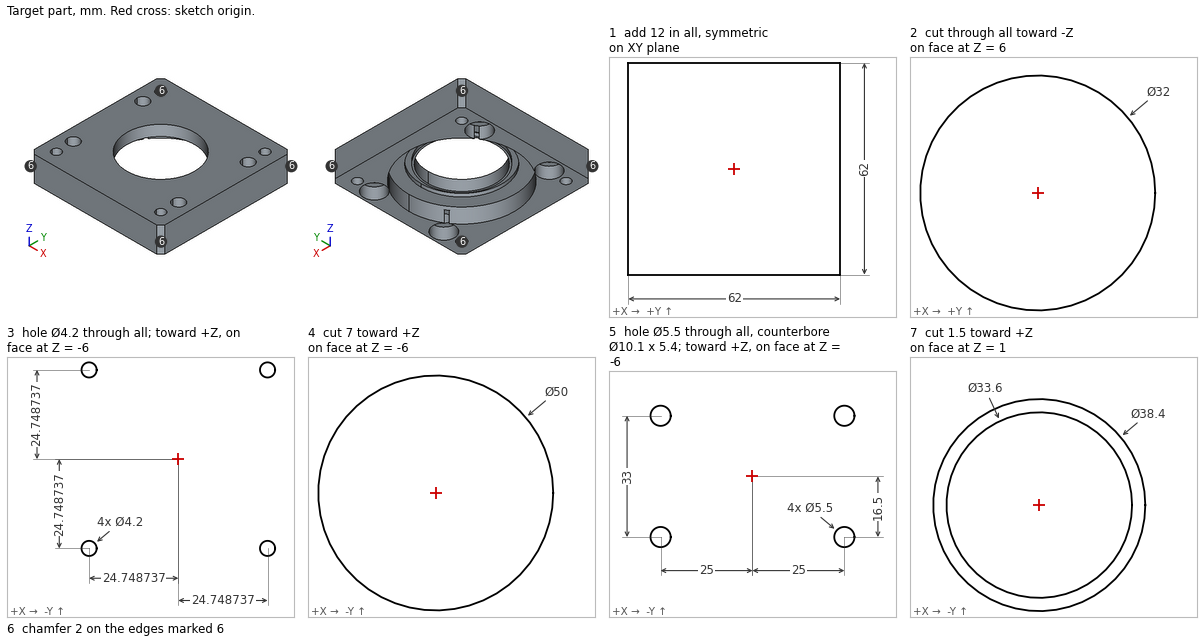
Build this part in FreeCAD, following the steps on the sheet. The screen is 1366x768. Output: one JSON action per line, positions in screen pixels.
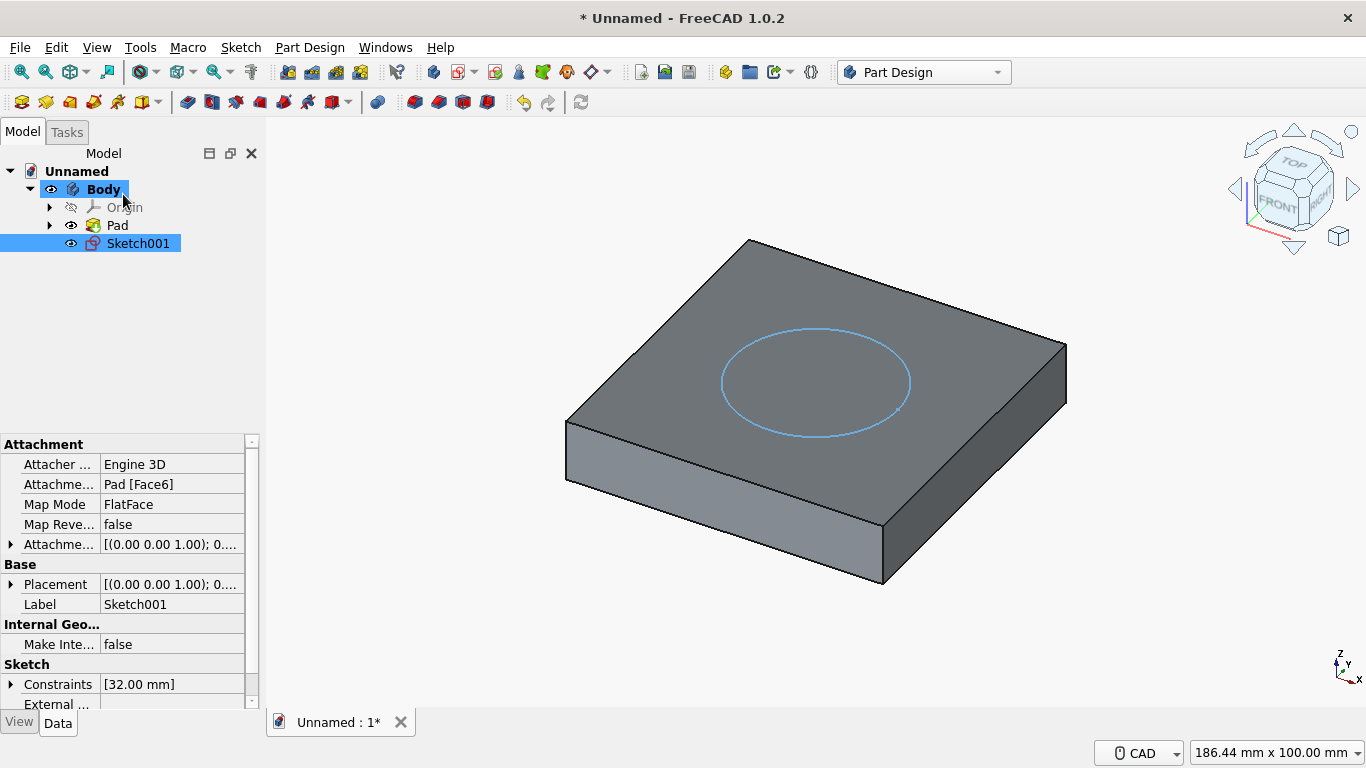
{"action": "left_click", "coordinate": [188, 102]}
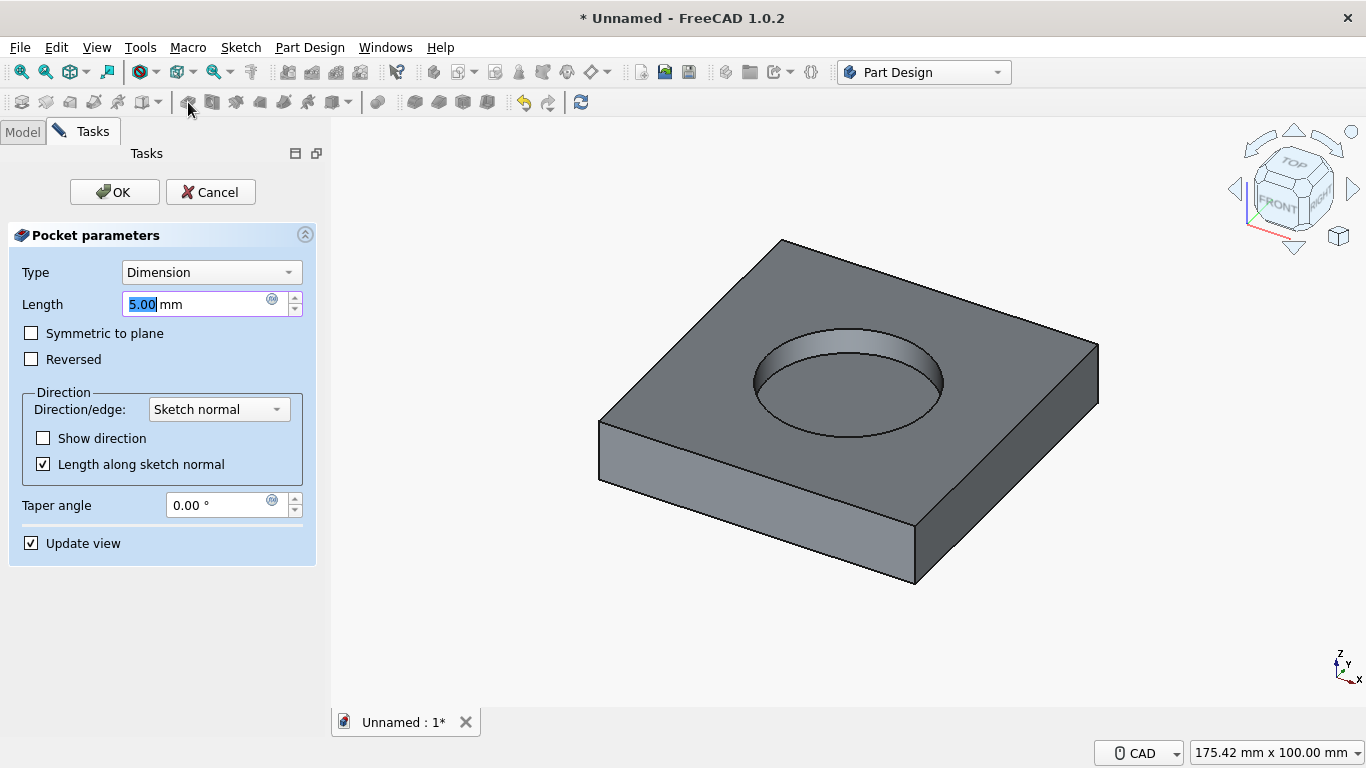
{"action": "left_click", "coordinate": [212, 272]}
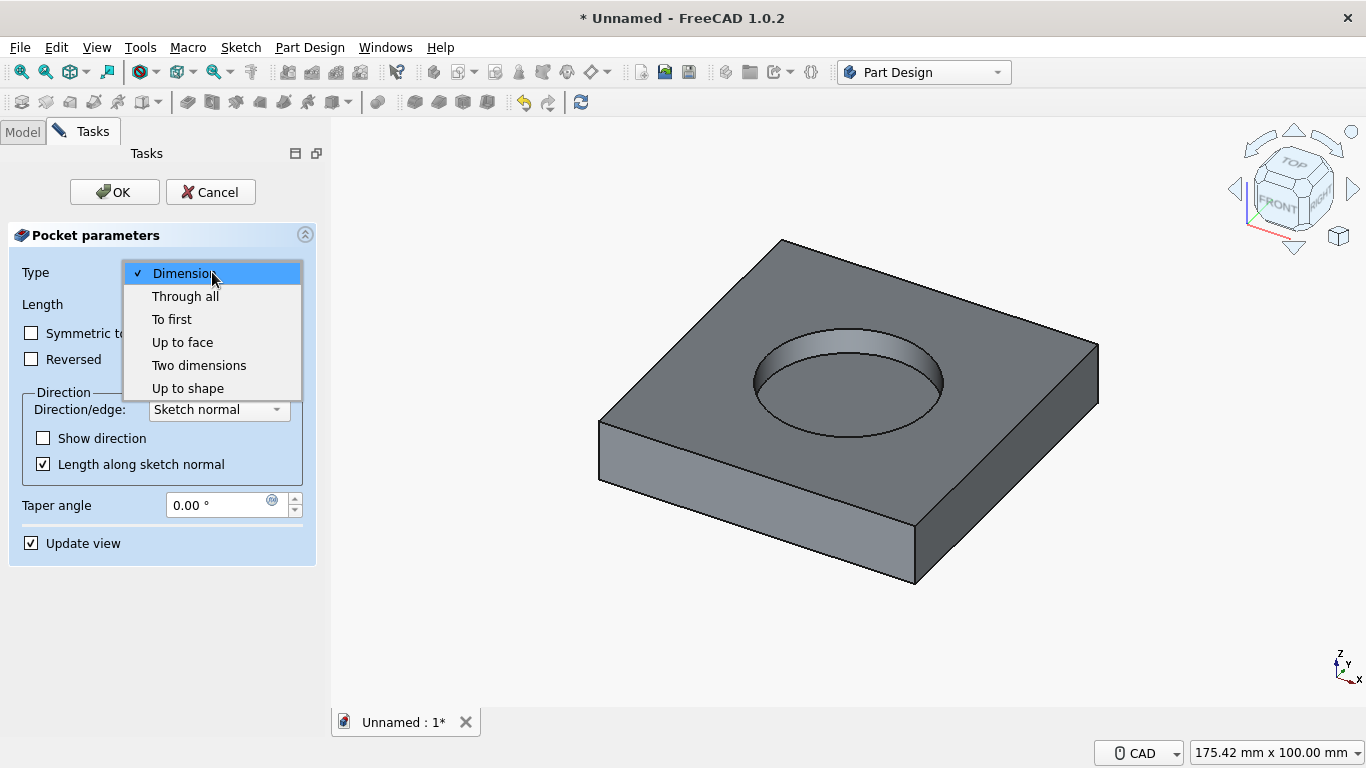
{"action": "left_click", "coordinate": [212, 296]}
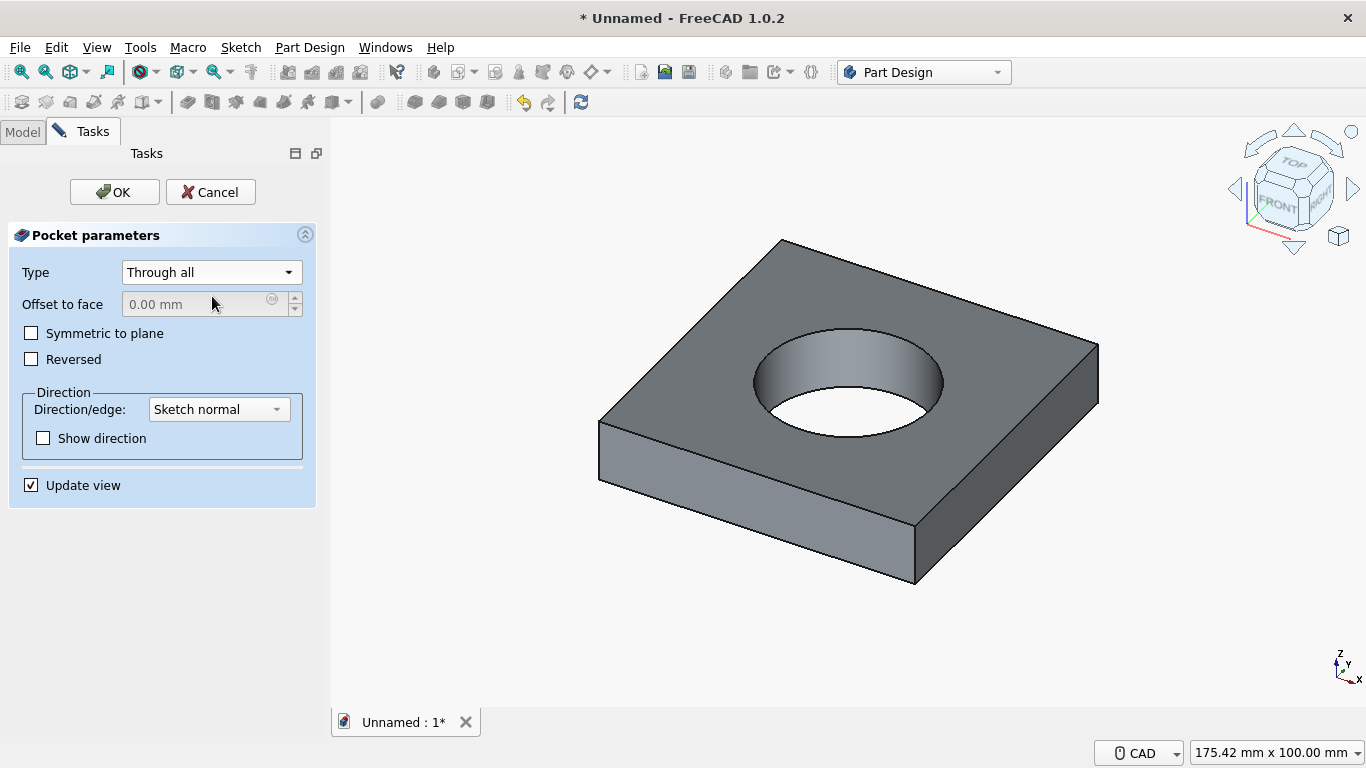
{"action": "left_click", "coordinate": [115, 192]}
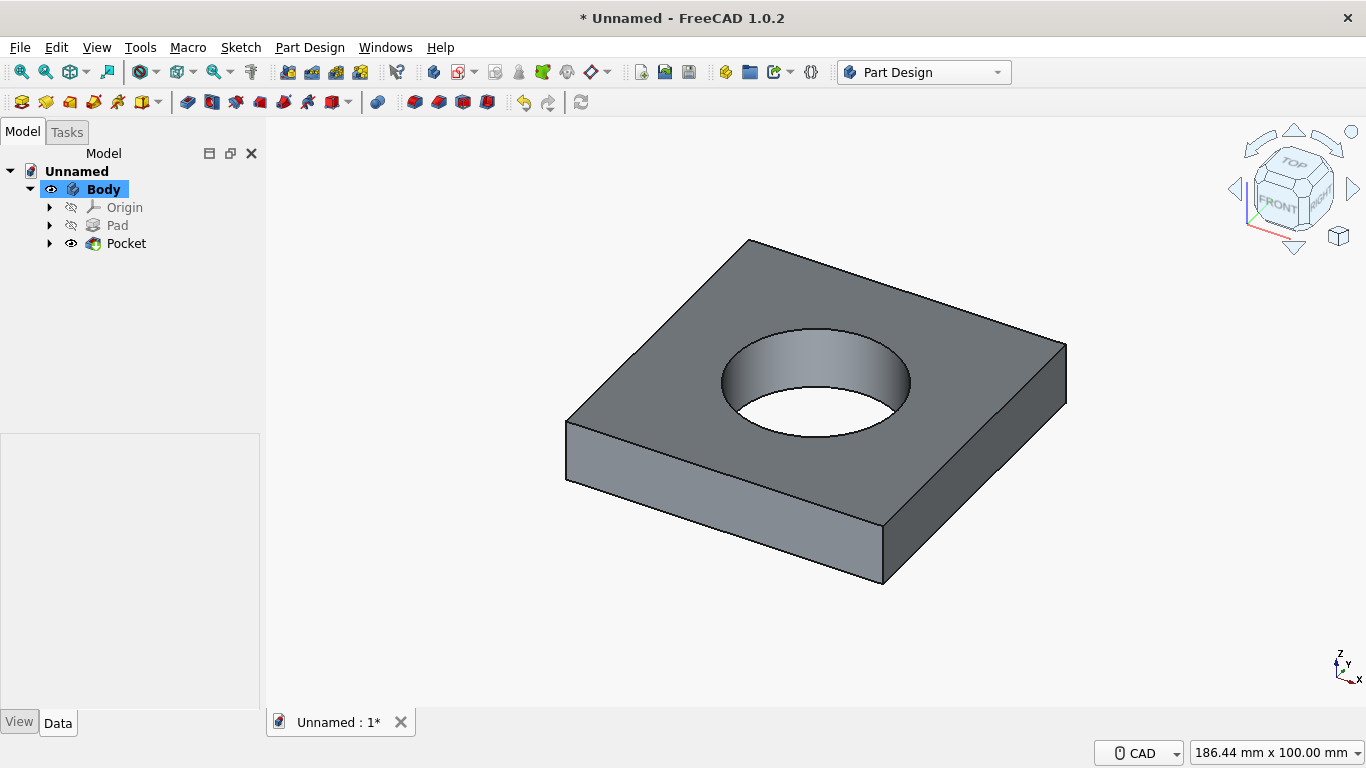
{"action": "key", "text": "5"}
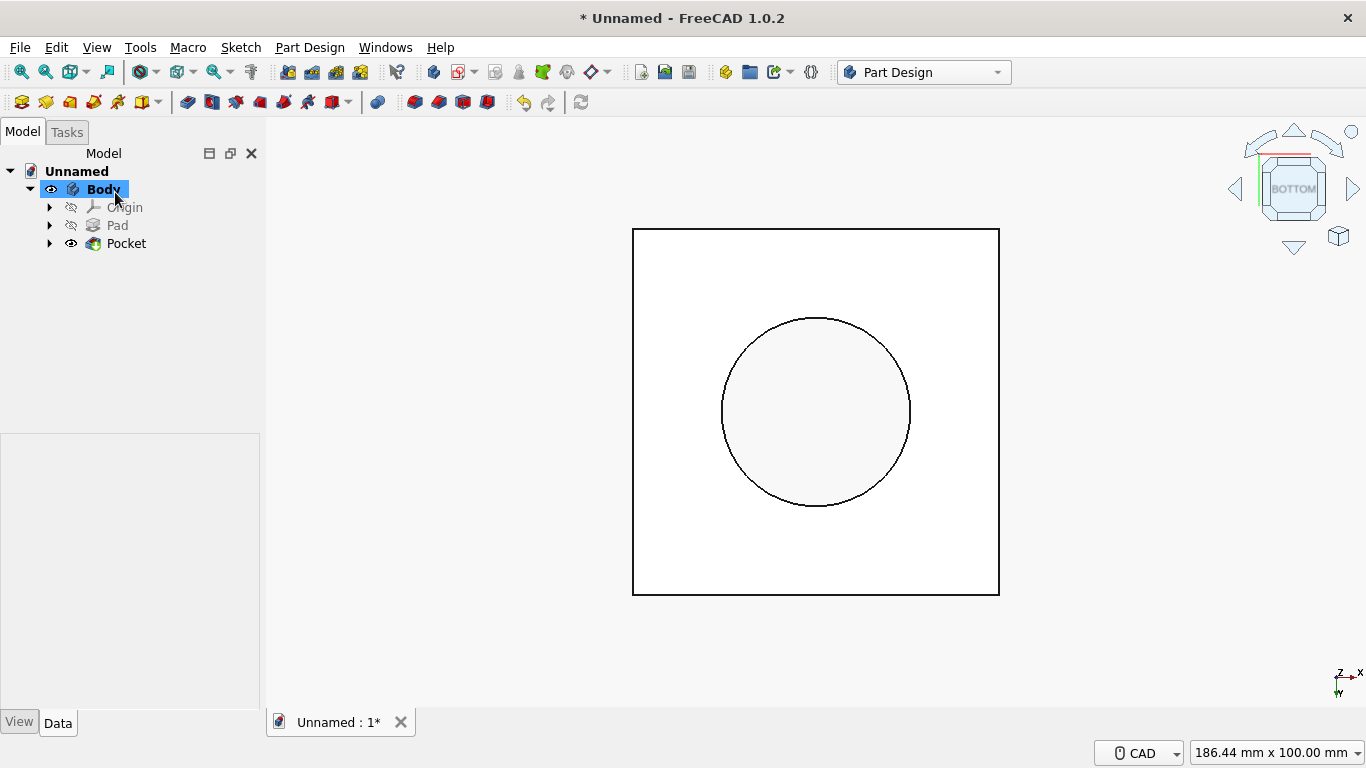
{"action": "left_click", "coordinate": [921, 516]}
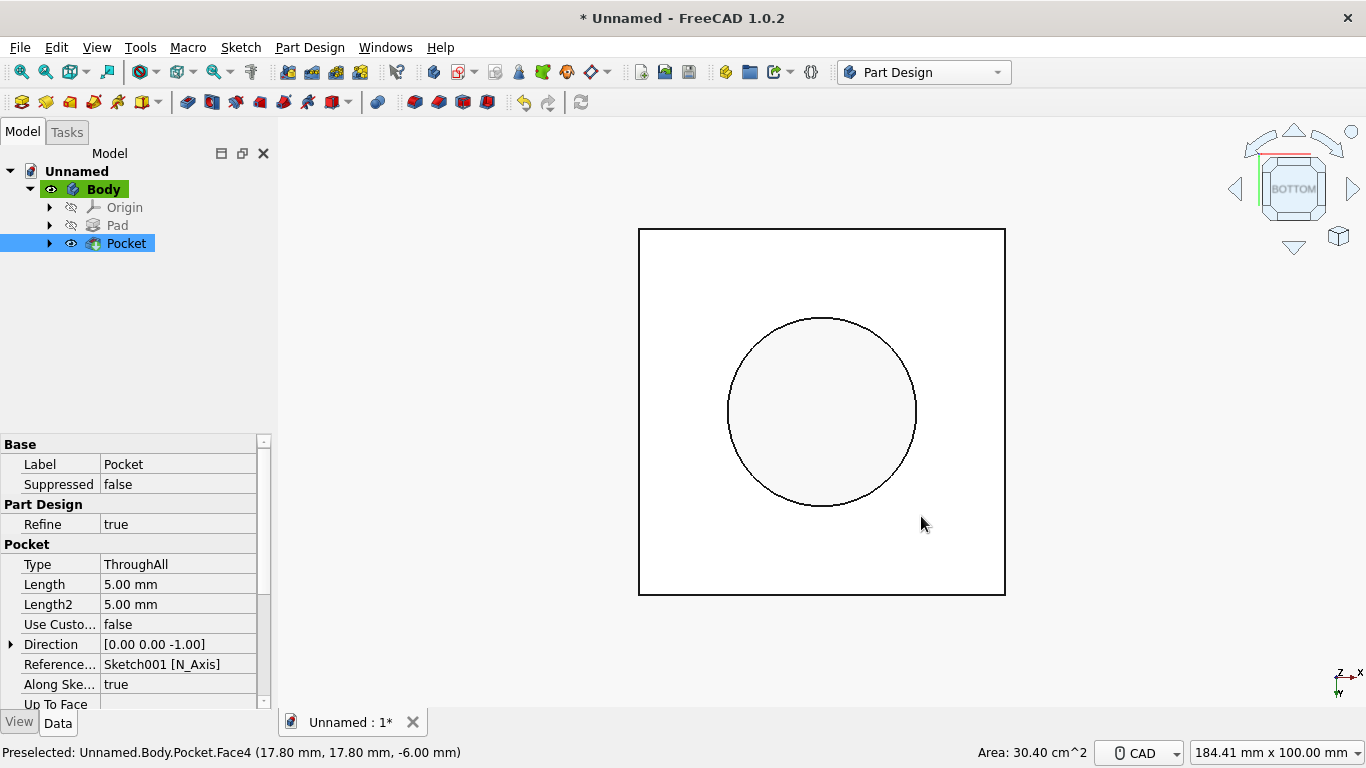
{"action": "left_click", "coordinate": [458, 72]}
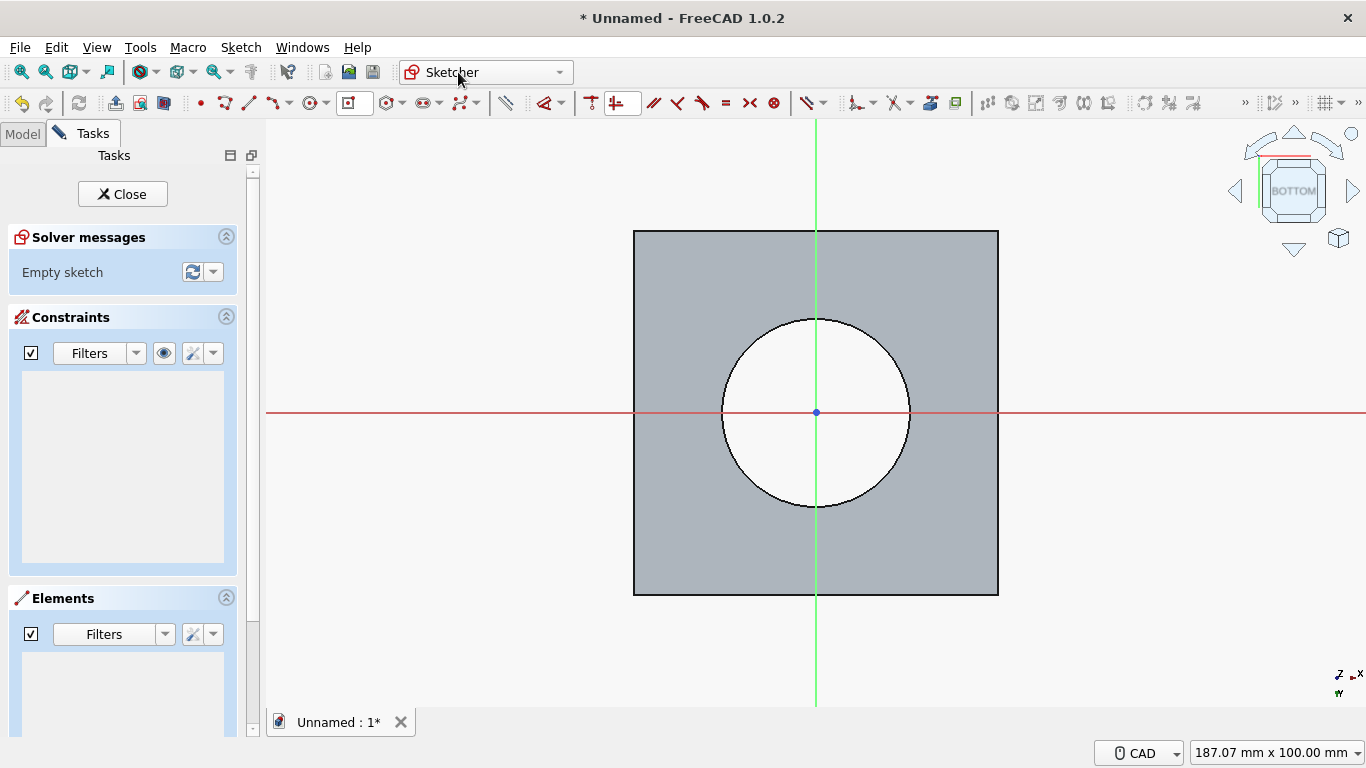
{"action": "left_click", "coordinate": [310, 104]}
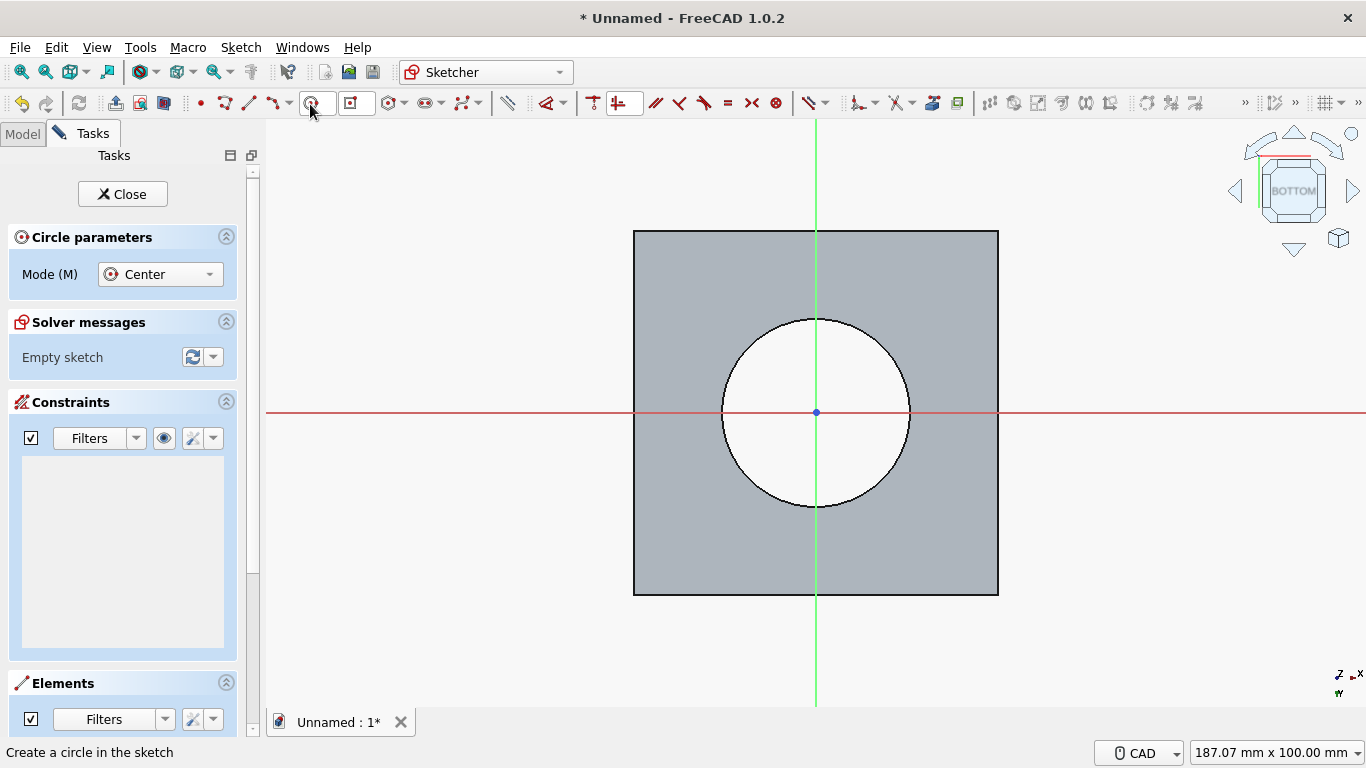
{"action": "scroll", "coordinate": [670, 559], "scroll_direction": "up", "scroll_amount": 4}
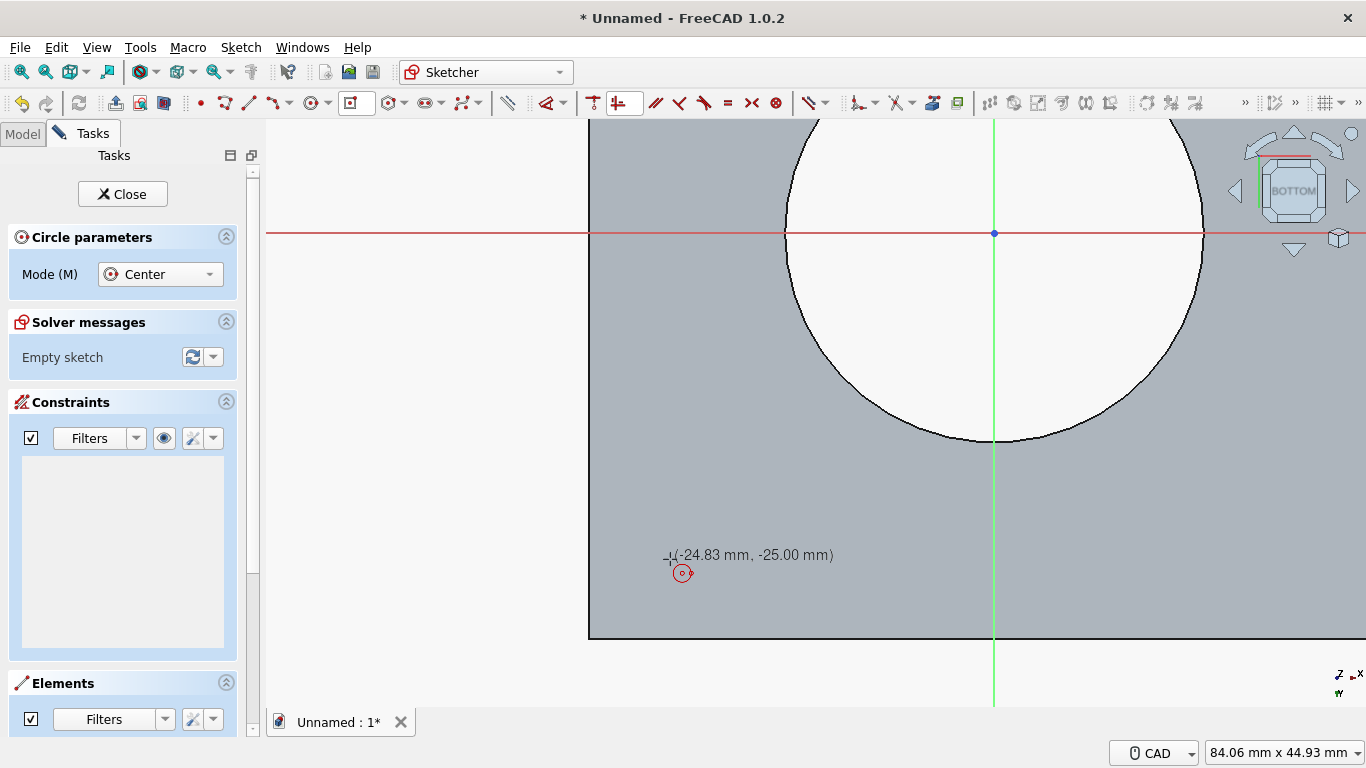
{"action": "left_click", "coordinate": [671, 557]}
{"action": "mouse_move", "coordinate": [690, 538]}